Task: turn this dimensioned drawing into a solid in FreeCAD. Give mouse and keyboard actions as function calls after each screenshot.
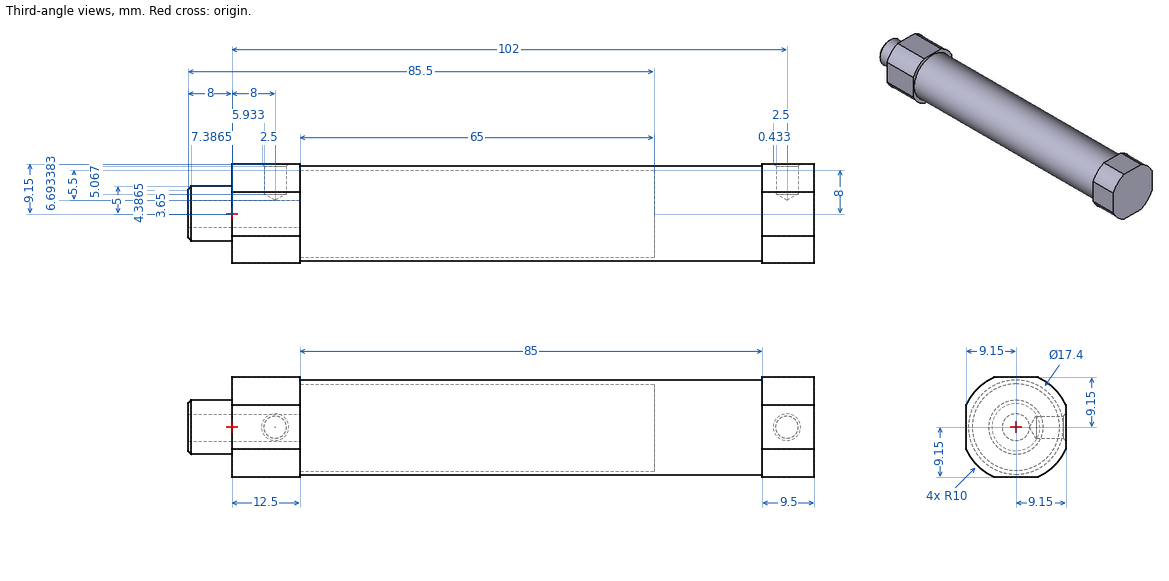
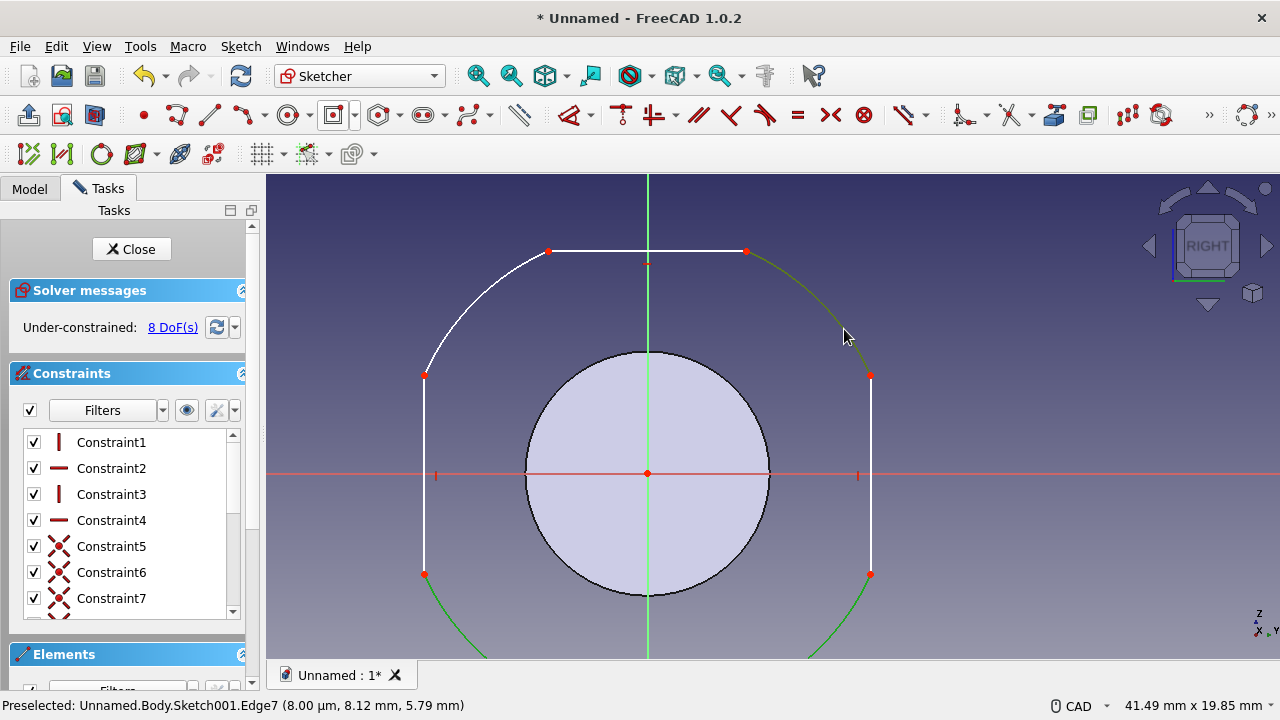
click(502, 278)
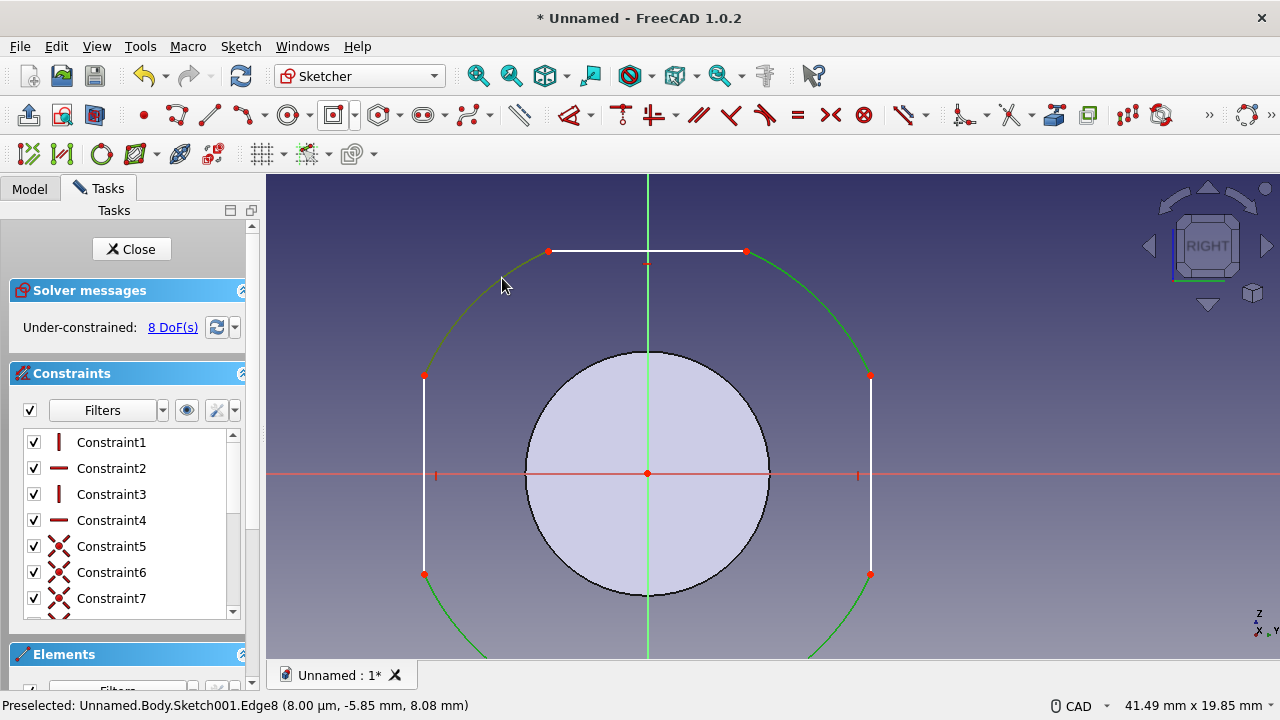
click(798, 116)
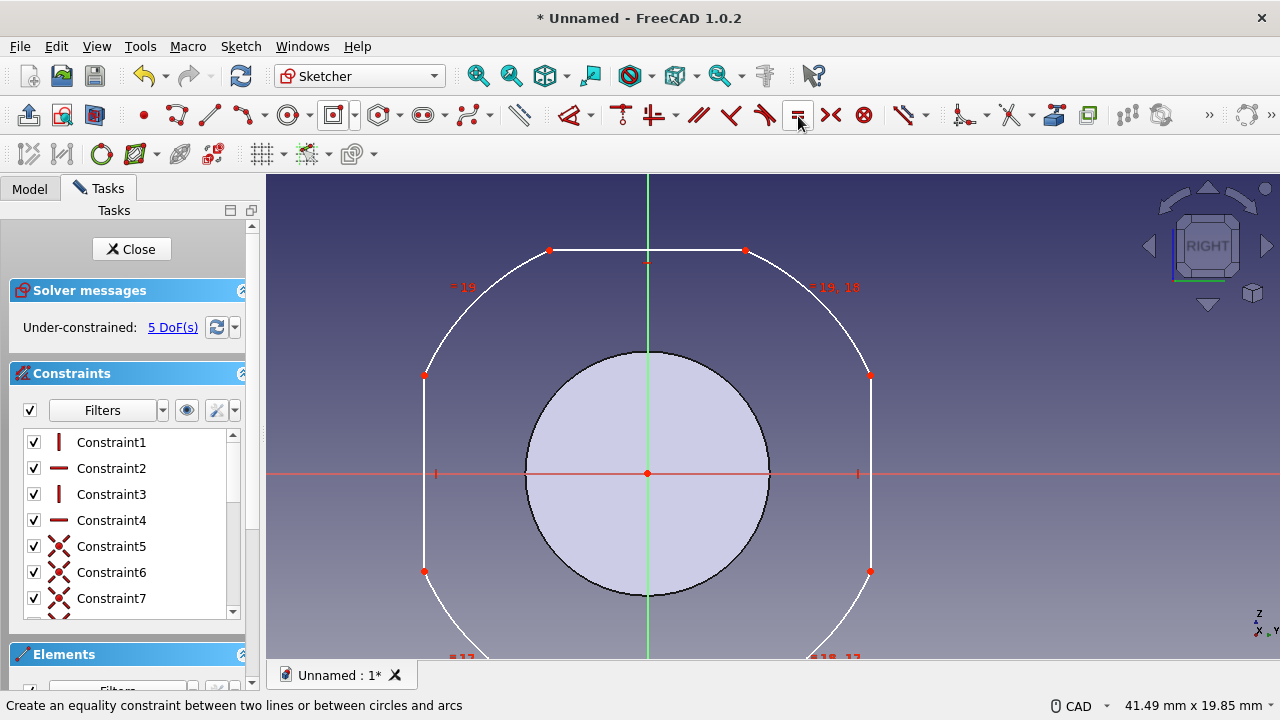
click(568, 116)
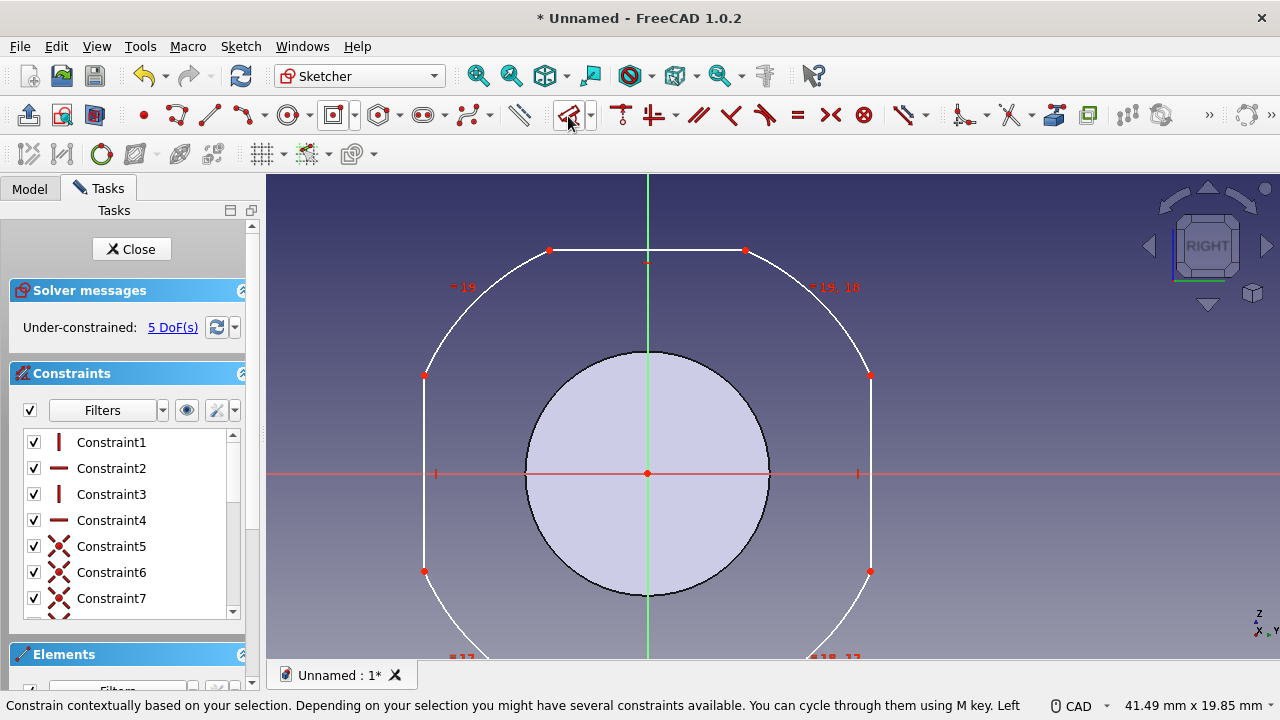
click(451, 618)
click(374, 510)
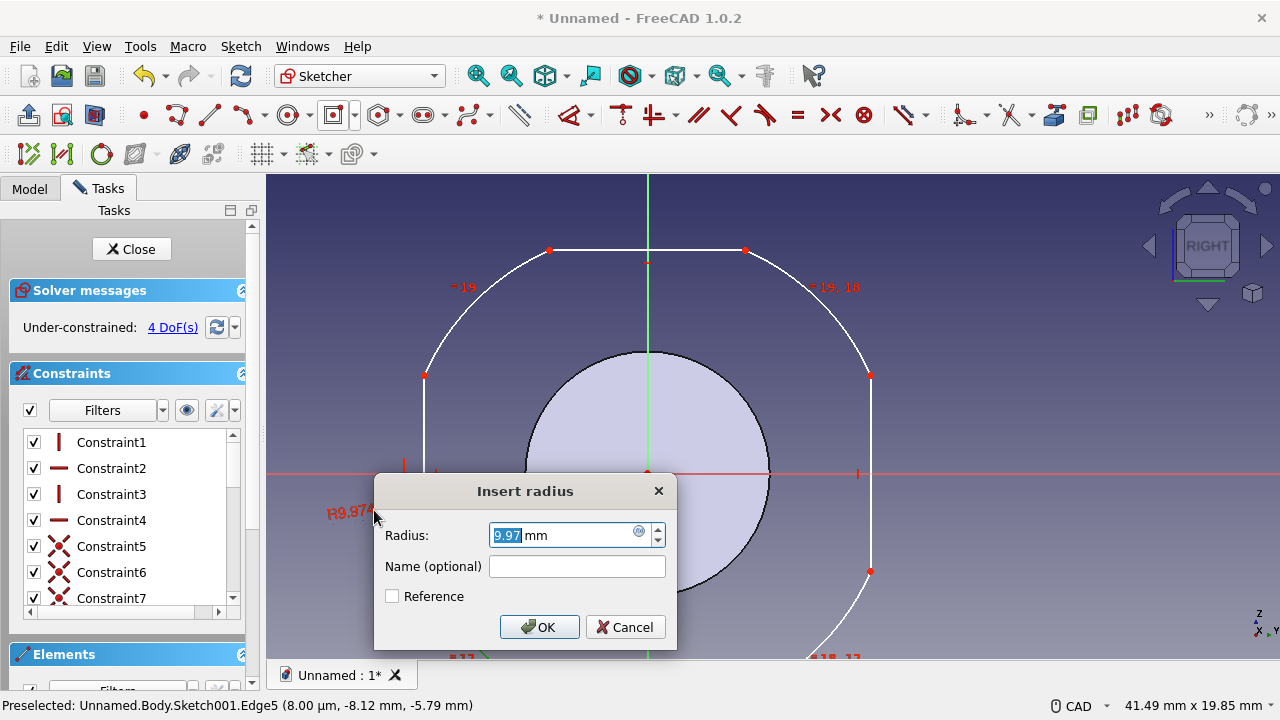
text(10)
key(Return)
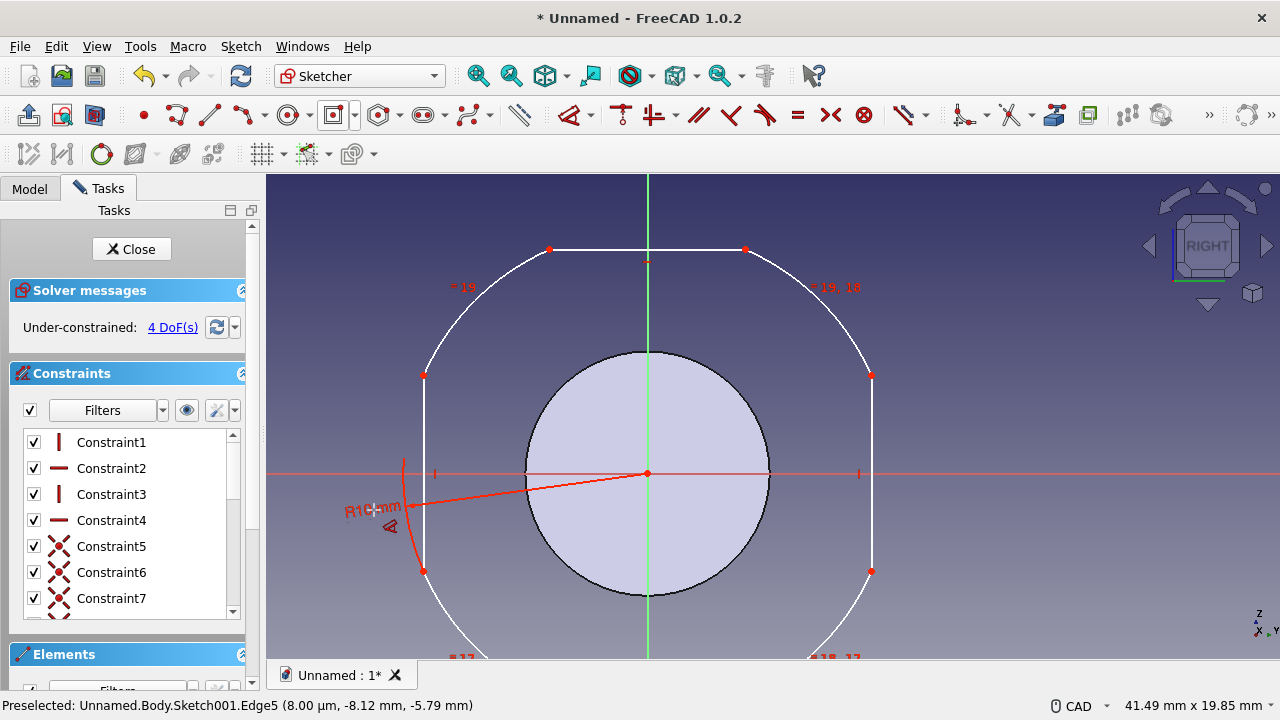
click(424, 376)
click(536, 342)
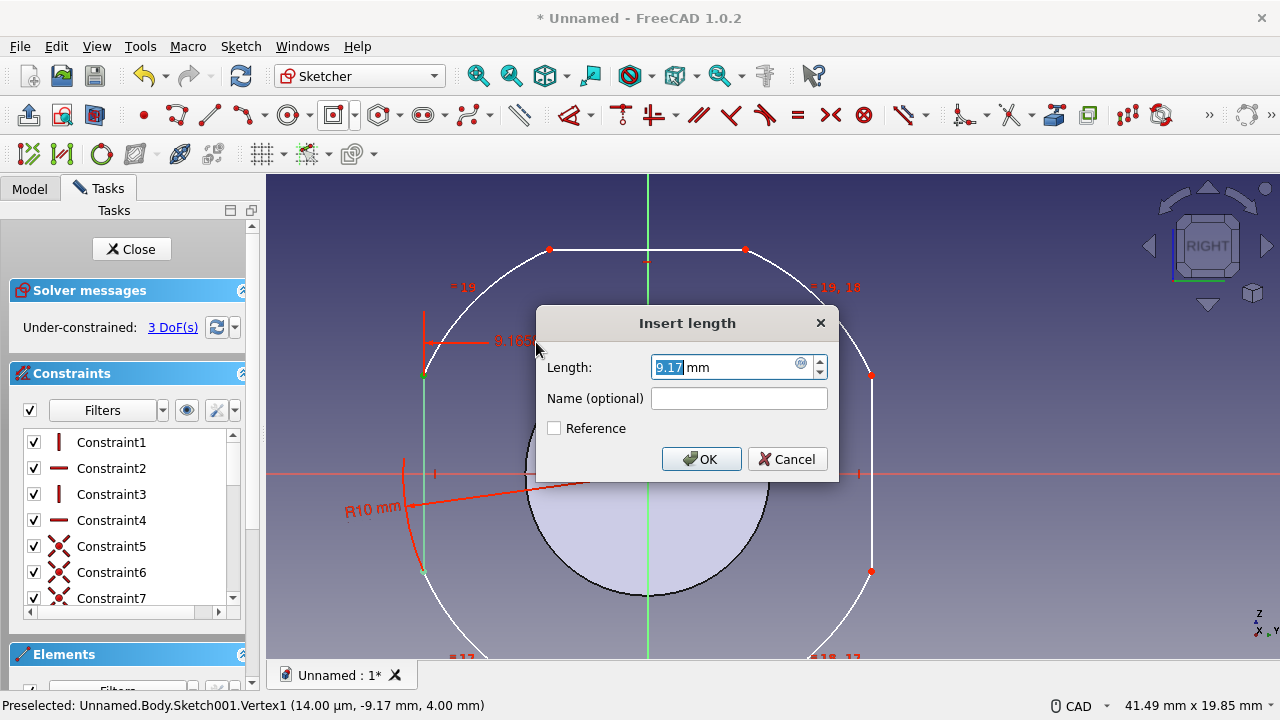
text(9.15)
key(Return)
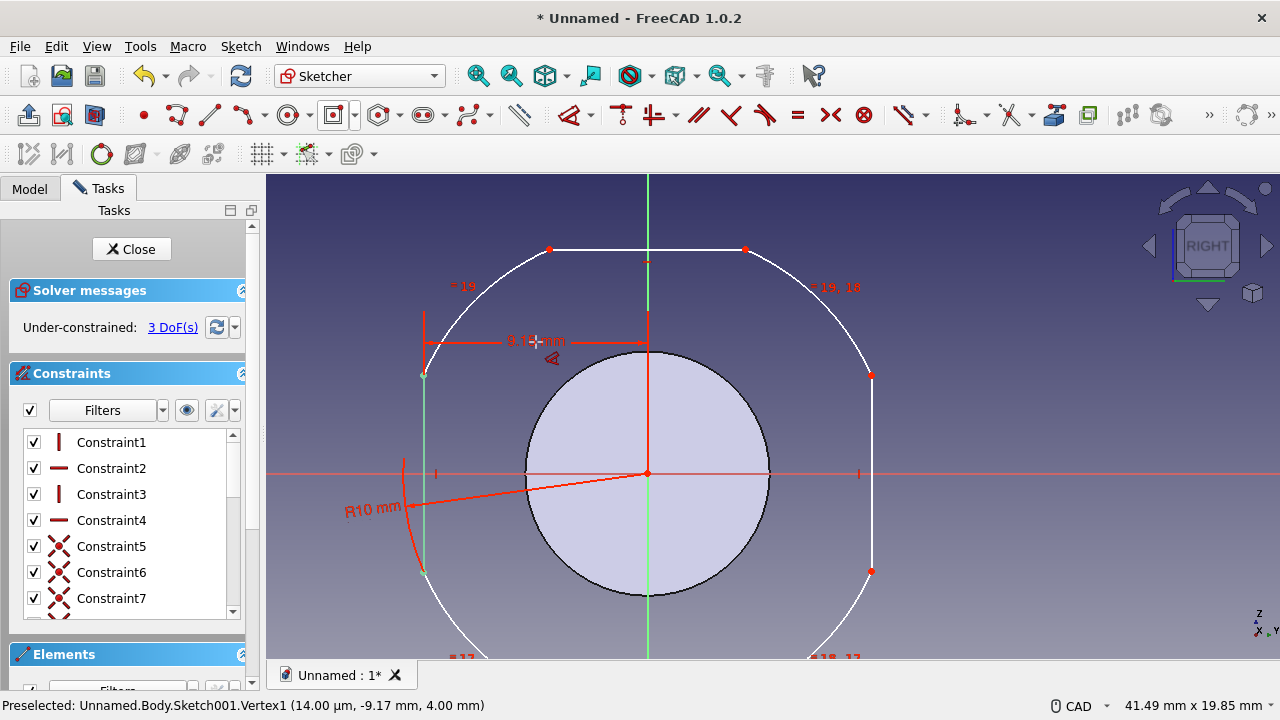
scroll(820, 300, down, 2)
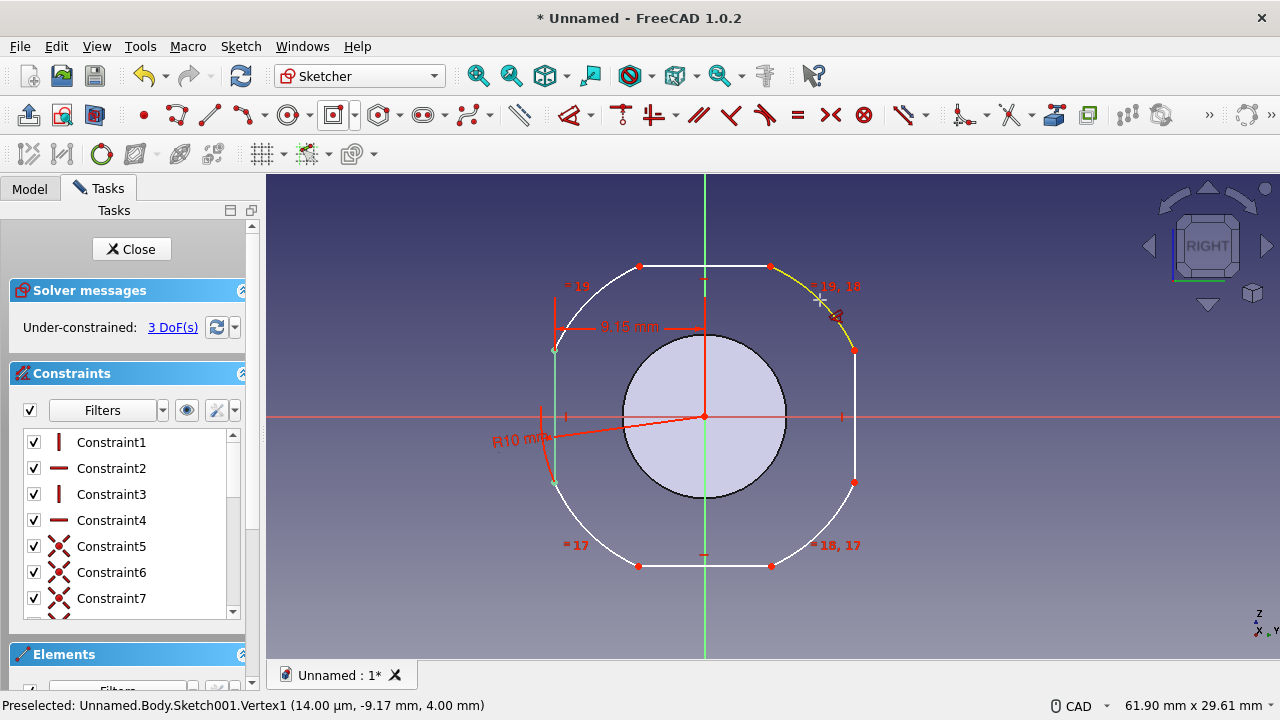
click(638, 566)
click(604, 491)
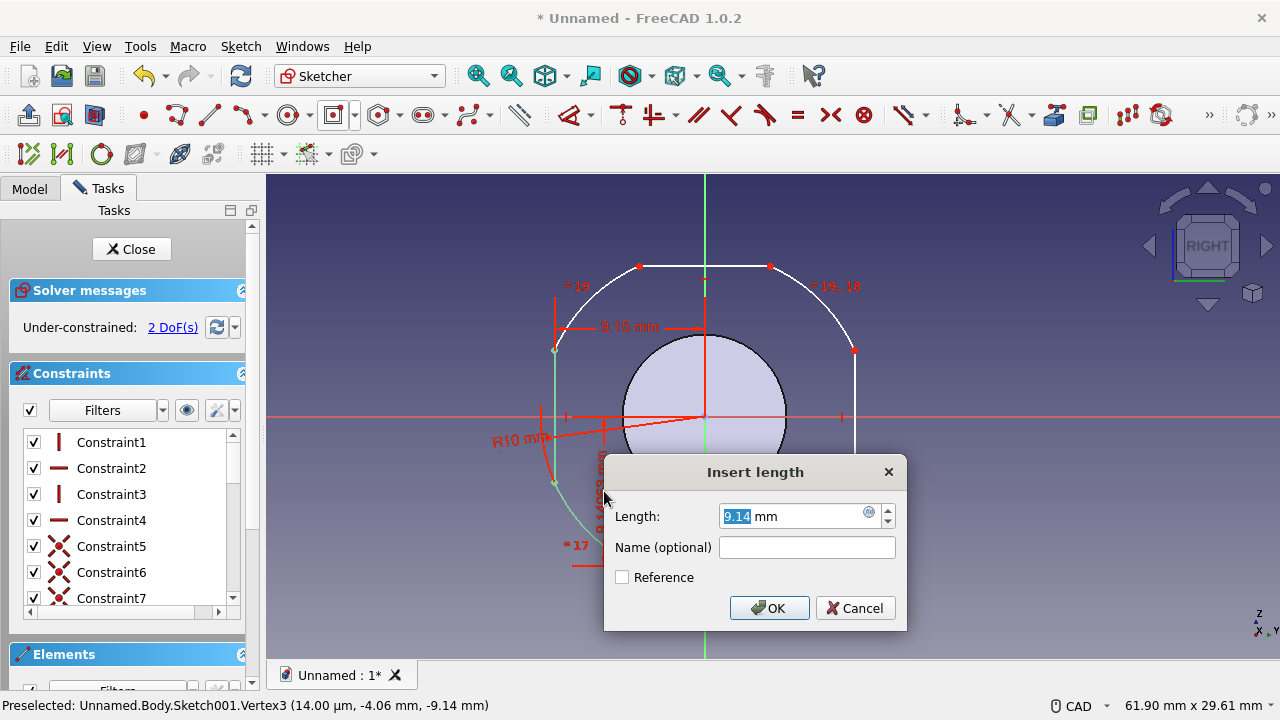
text(9.15)
key(Return)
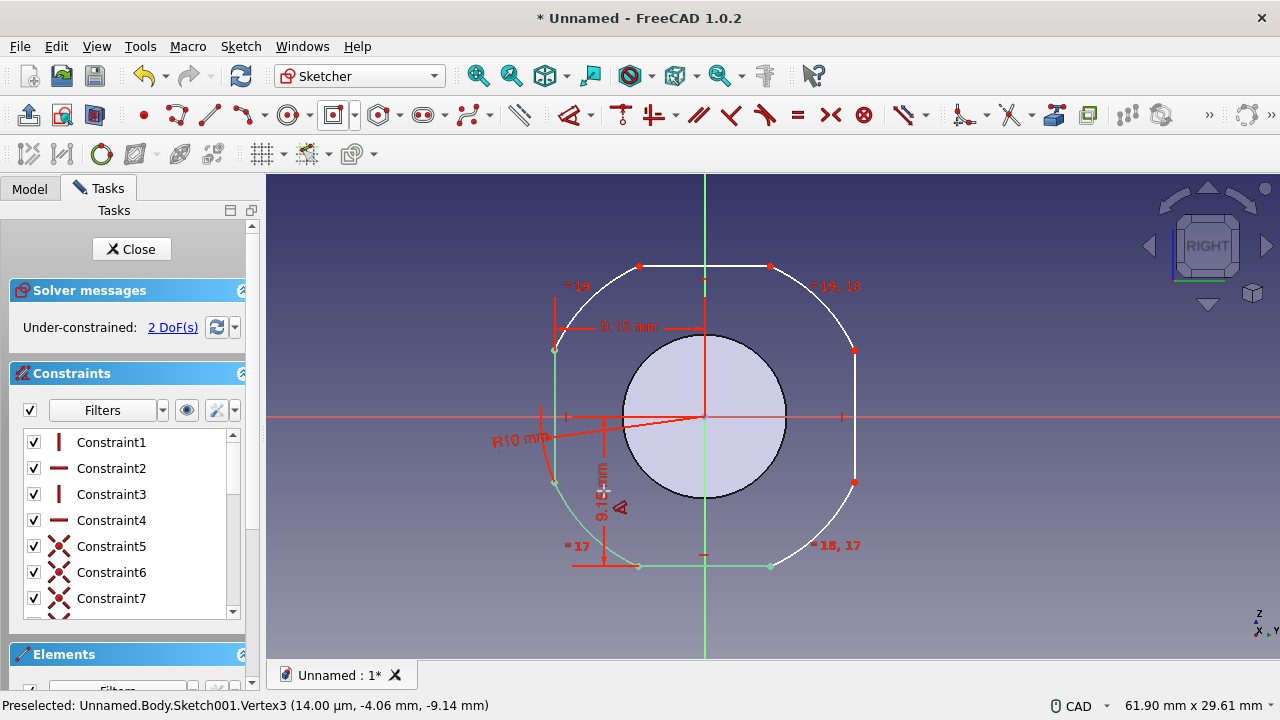
click(855, 482)
click(780, 516)